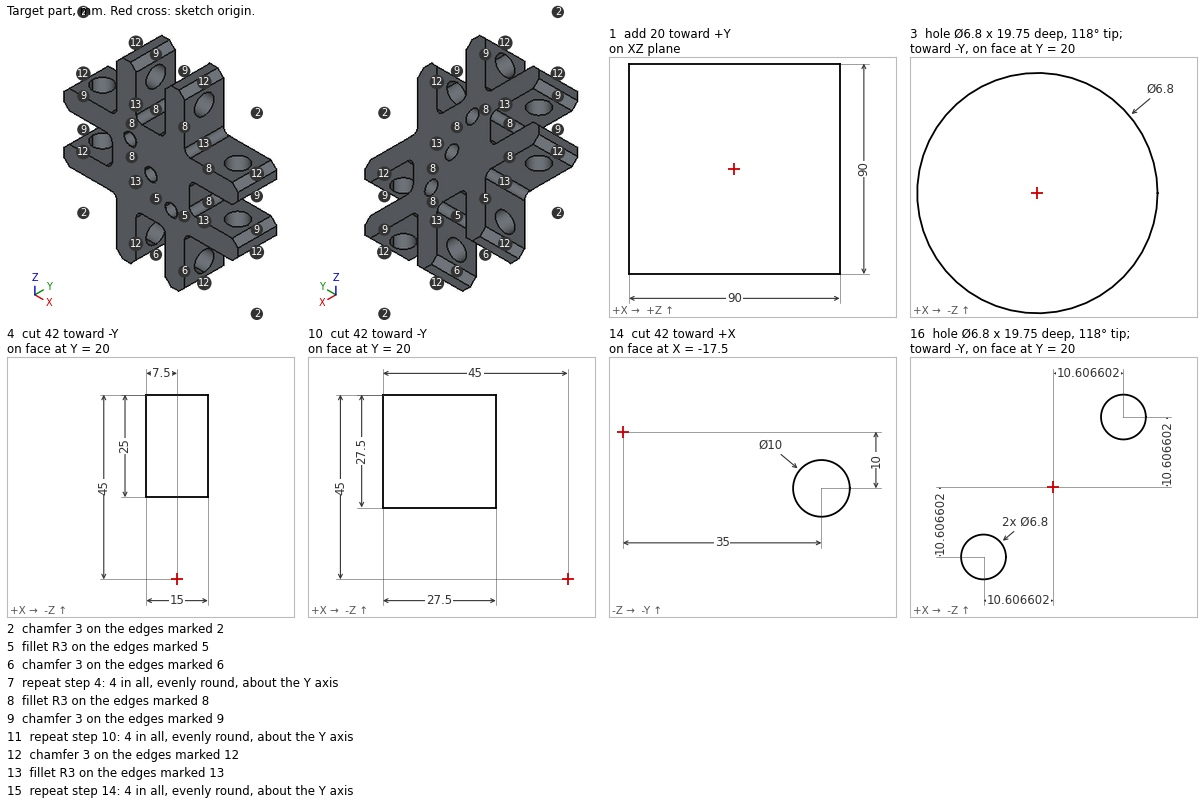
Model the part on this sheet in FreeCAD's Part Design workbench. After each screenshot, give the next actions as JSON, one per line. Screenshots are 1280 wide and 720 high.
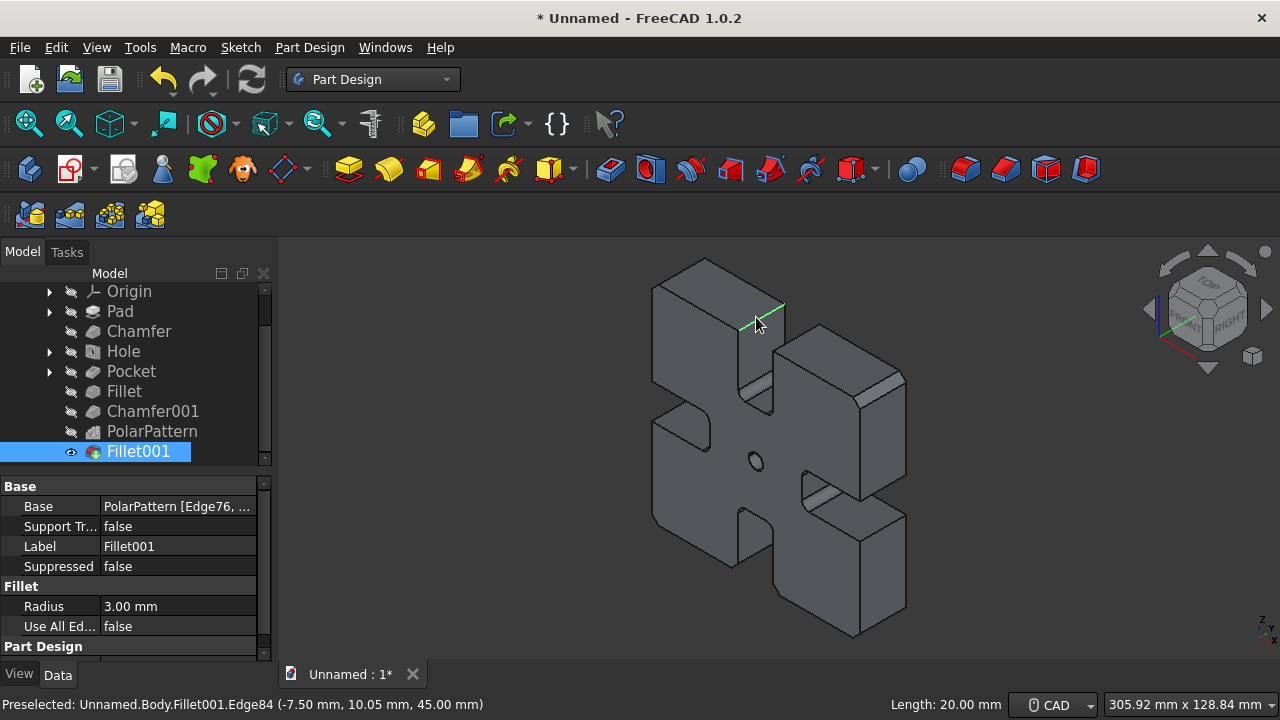
{"action": "left_click", "coordinate": [883, 527], "text": "ctrl"}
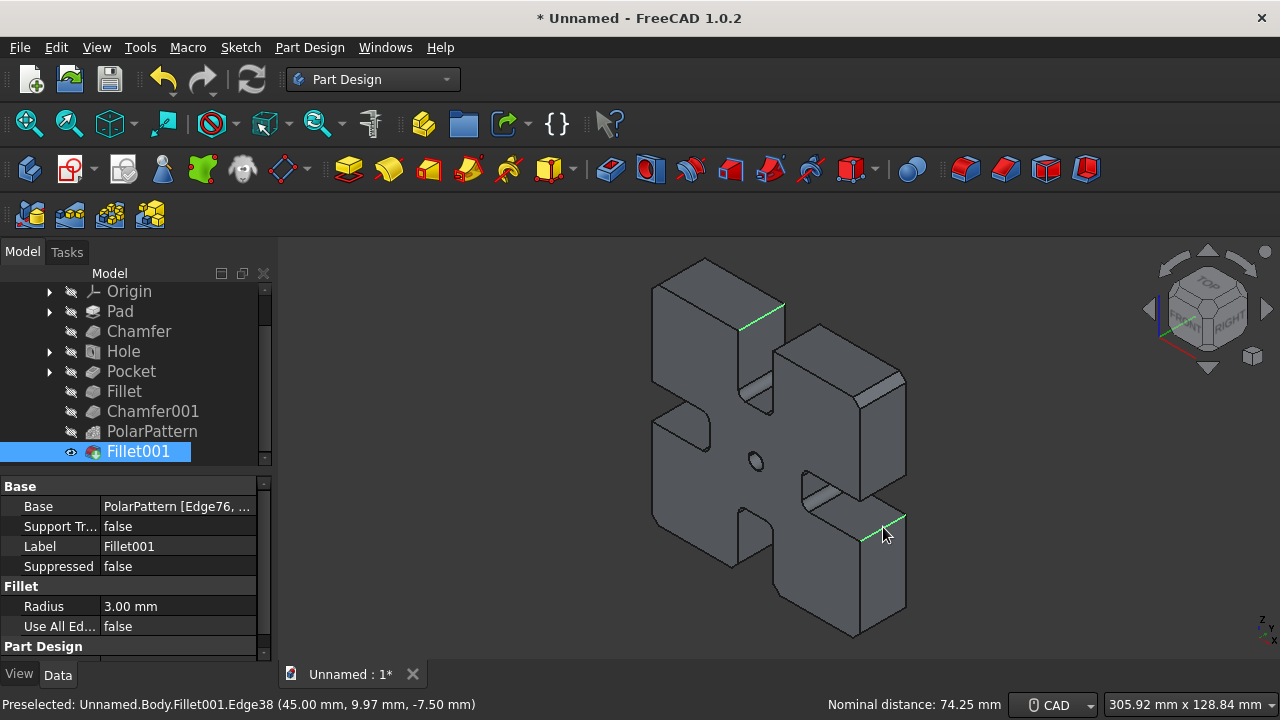
{"action": "key", "text": "2"}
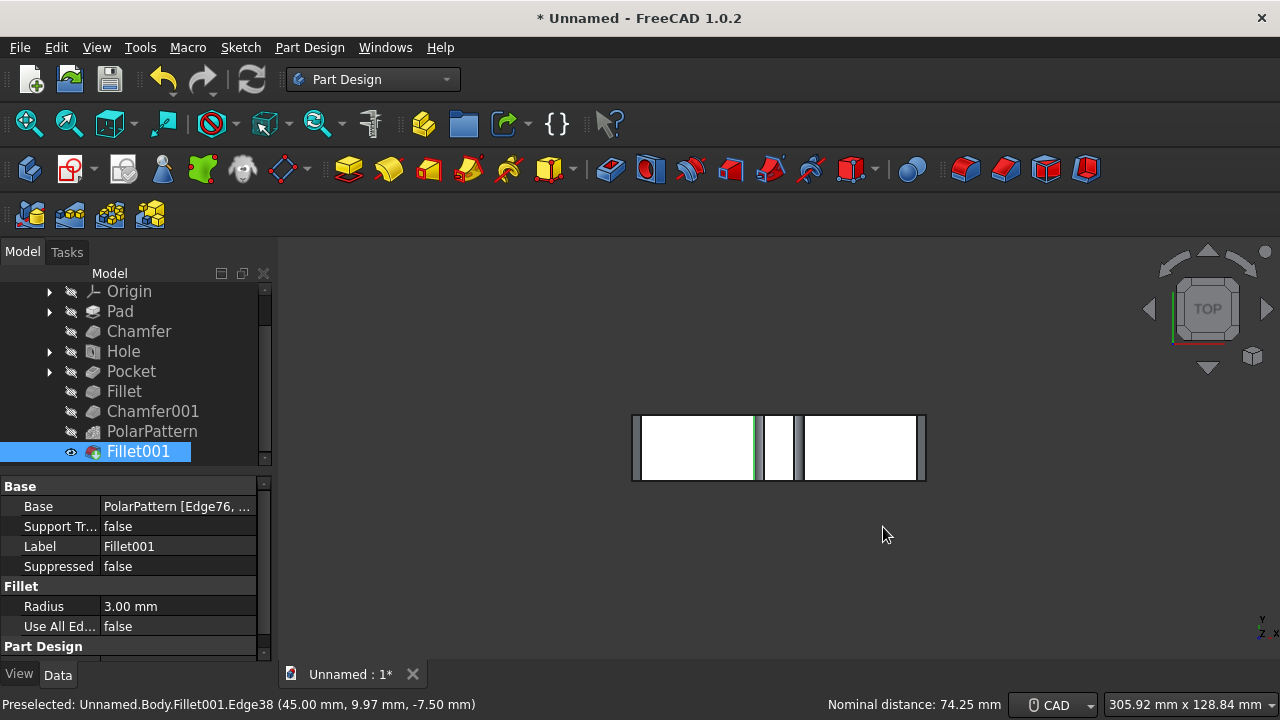
{"action": "left_click", "coordinate": [30, 124]}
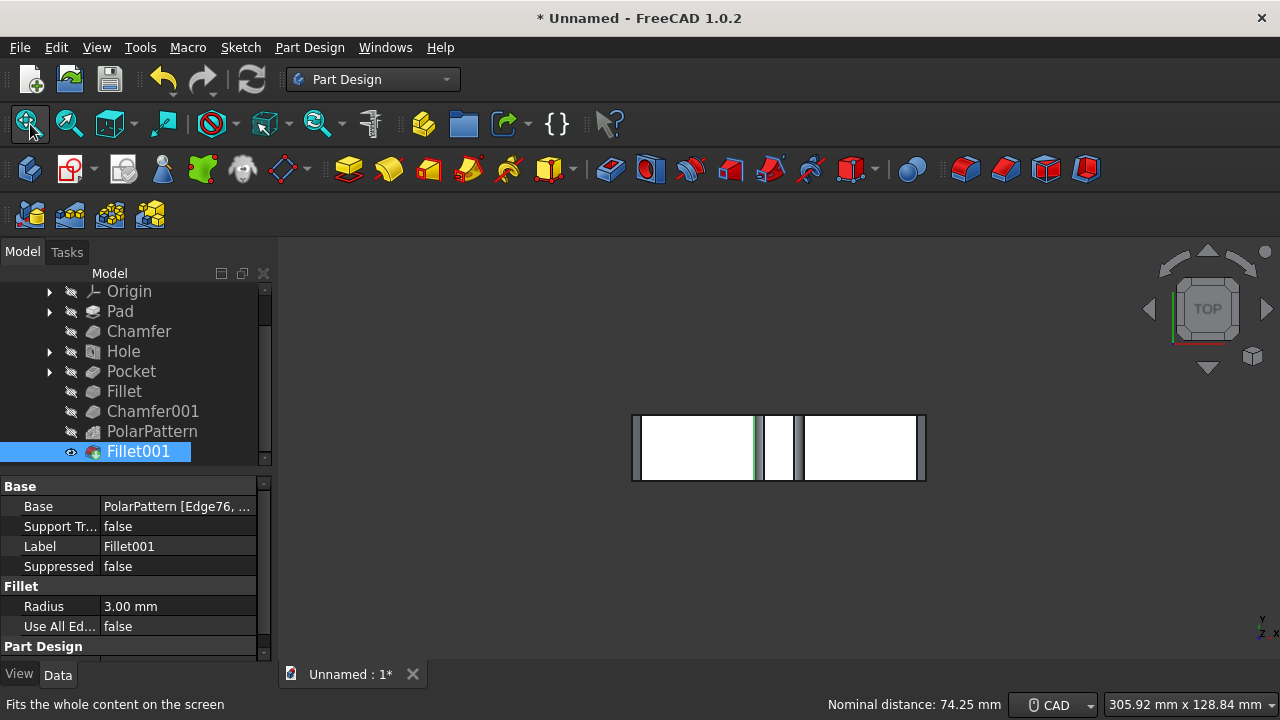
{"action": "left_click", "coordinate": [804, 447], "text": "ctrl"}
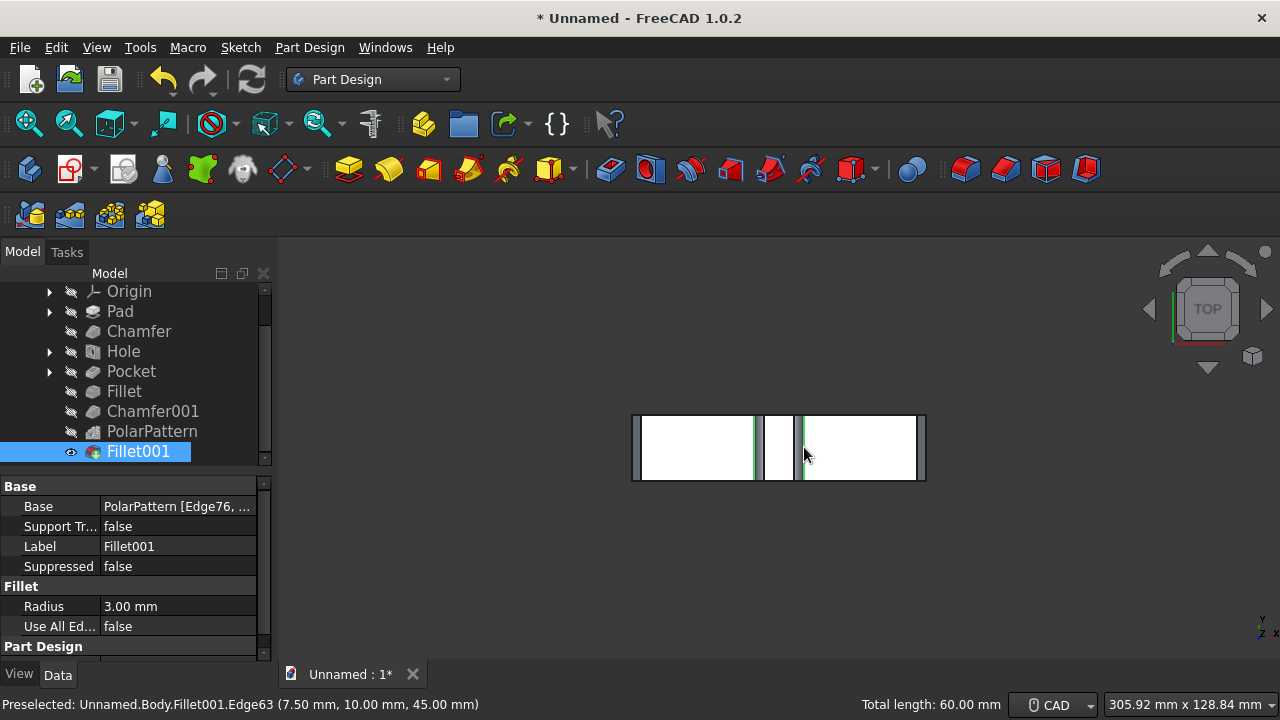
{"action": "key", "text": "0"}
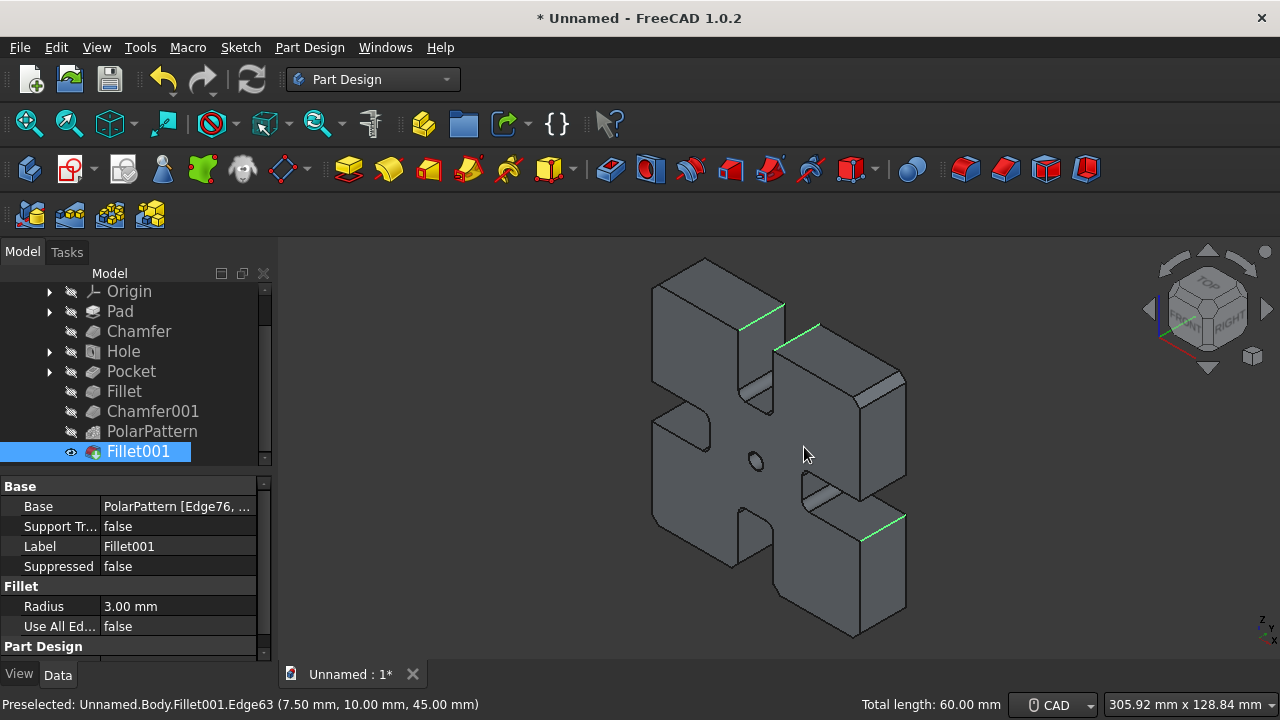
{"action": "key", "text": "1"}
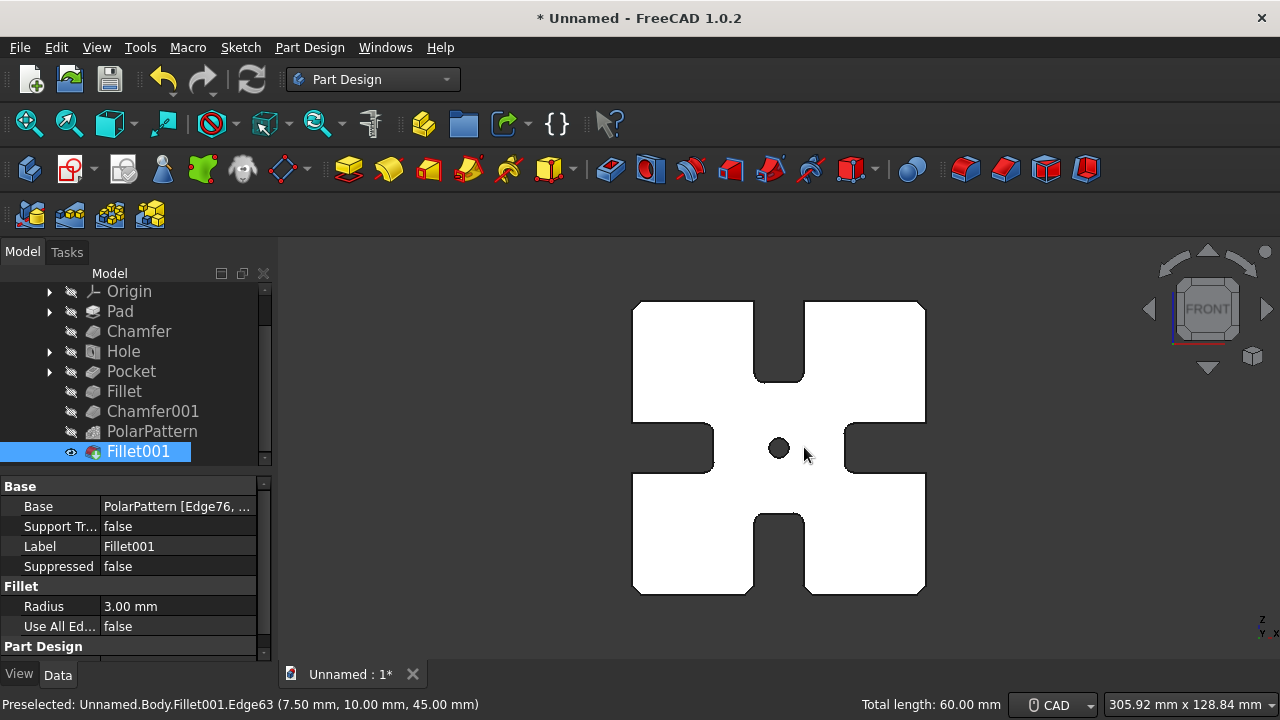
{"action": "key", "text": "3"}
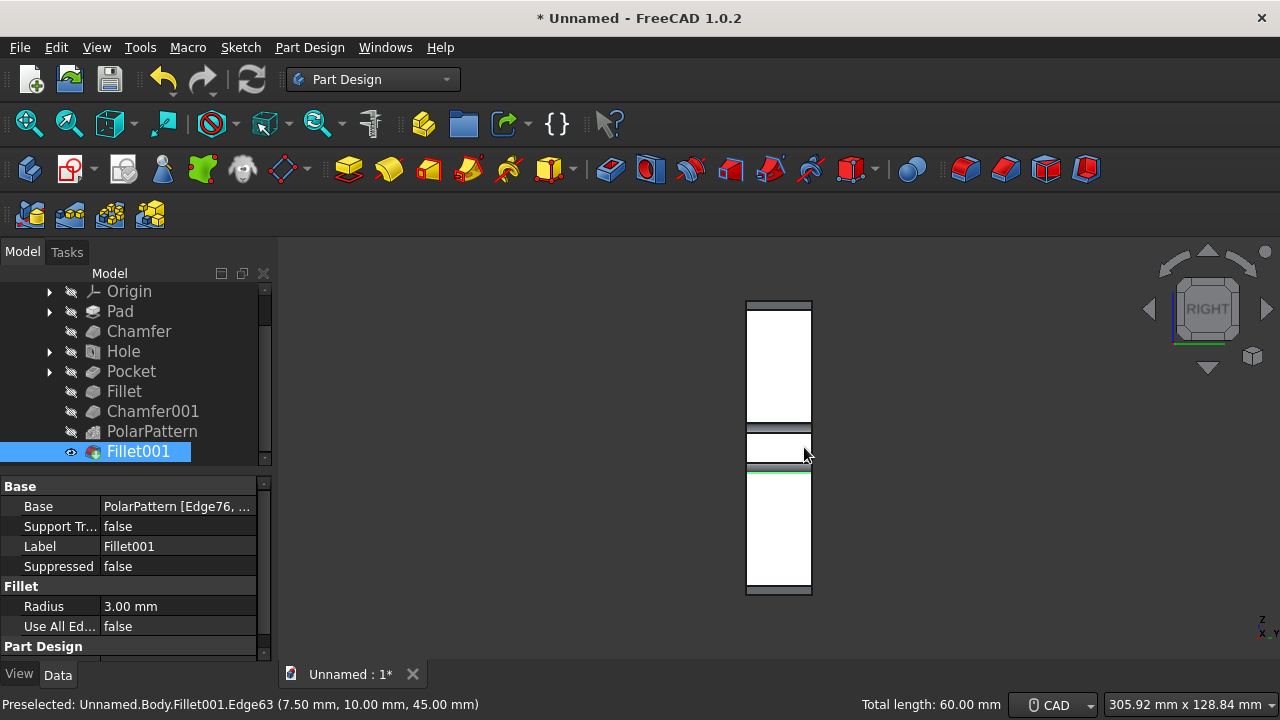
{"action": "left_click", "coordinate": [779, 422], "text": "ctrl"}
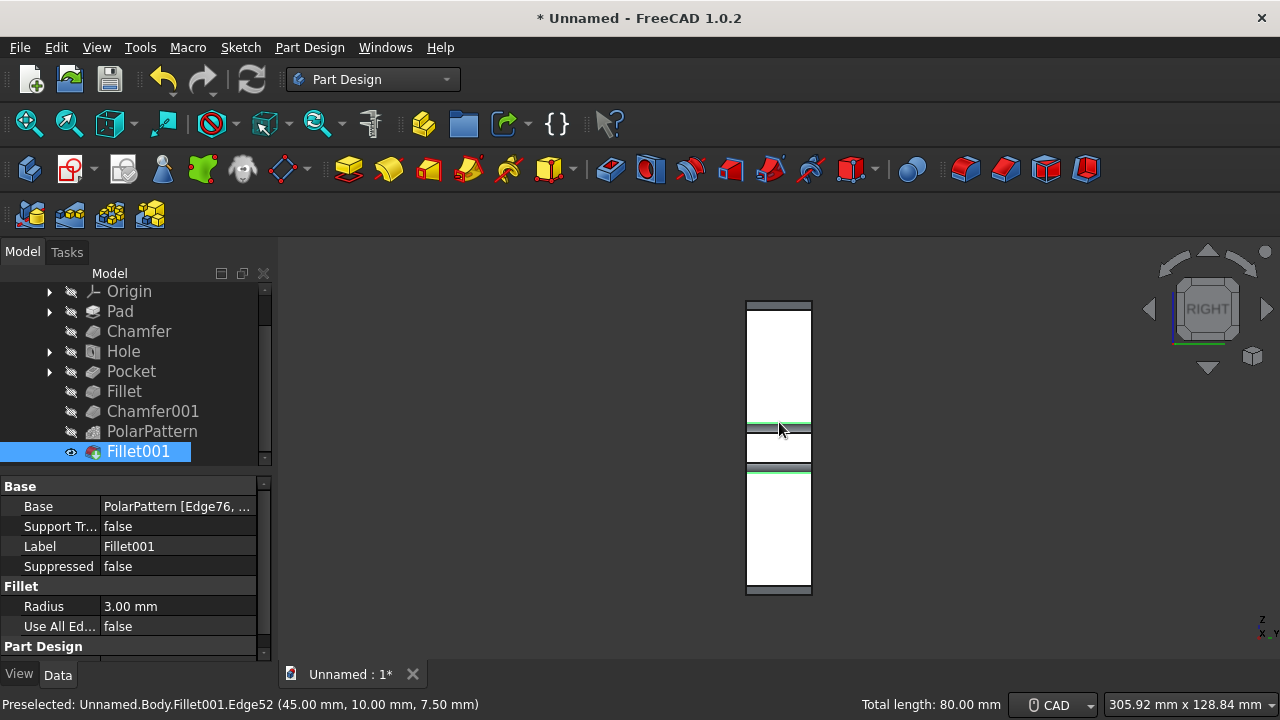
{"action": "key", "text": "5"}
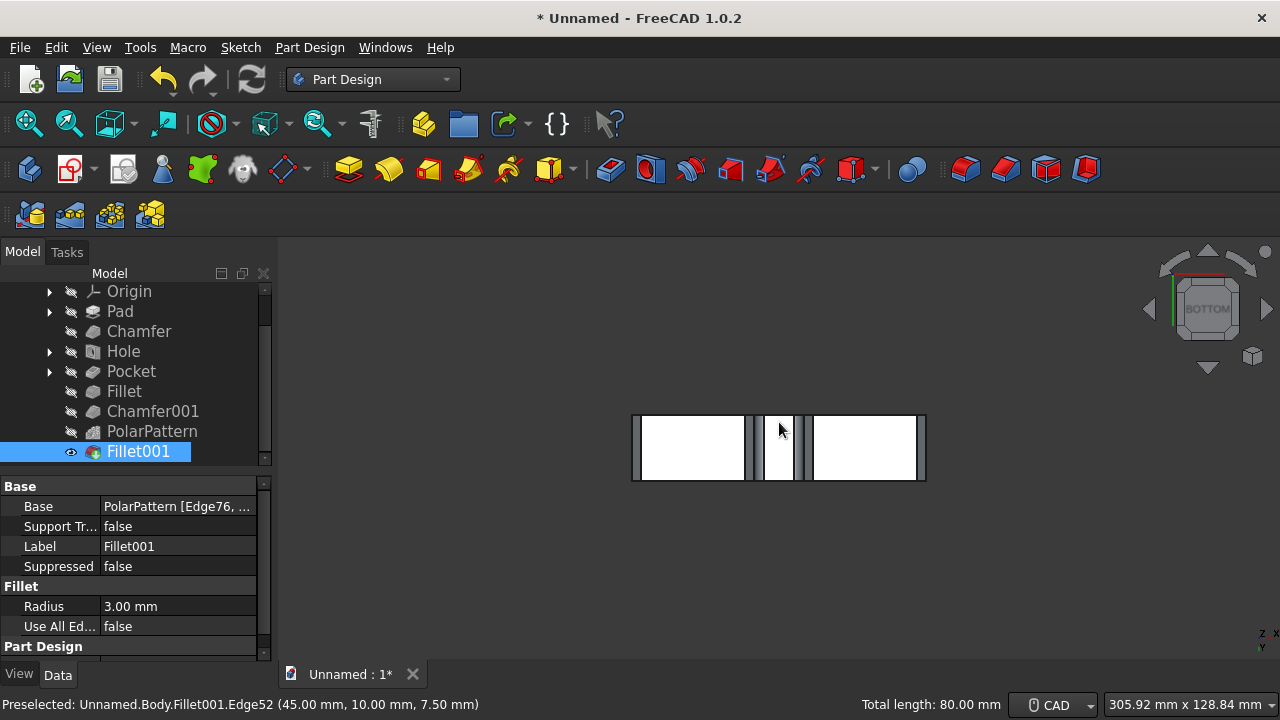
{"action": "left_click", "coordinate": [30, 124]}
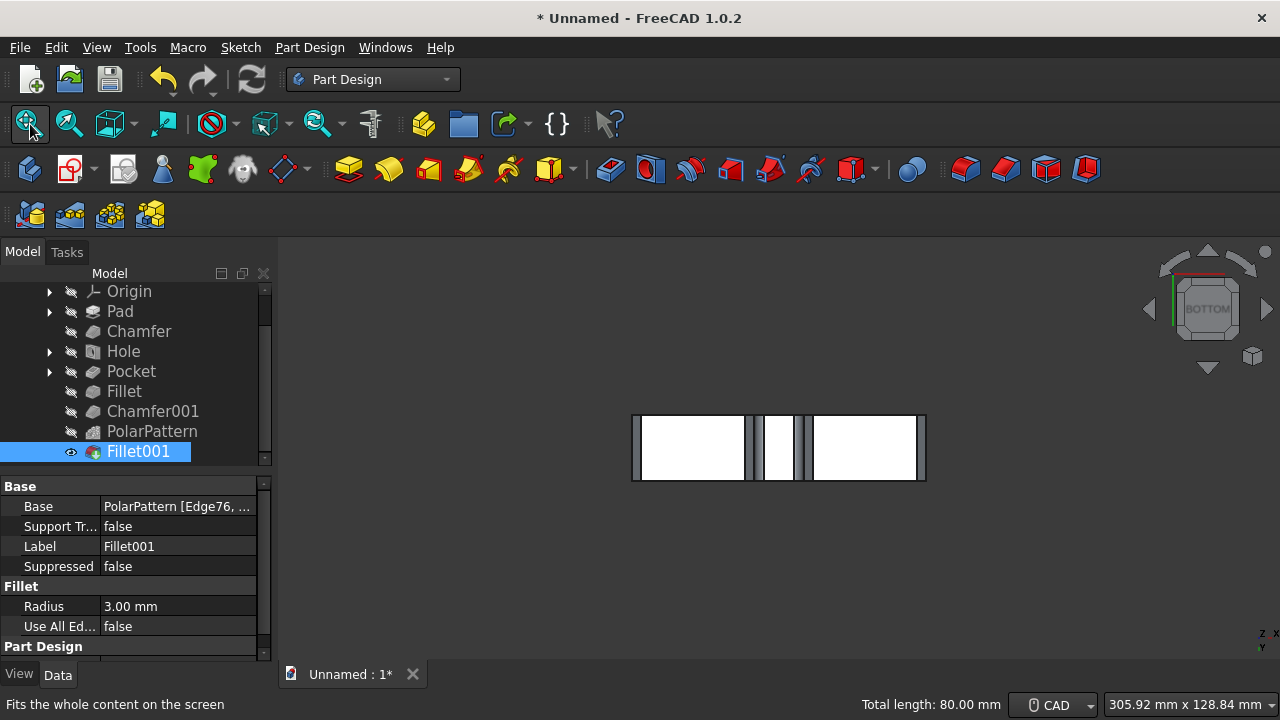
{"action": "key", "text": "4"}